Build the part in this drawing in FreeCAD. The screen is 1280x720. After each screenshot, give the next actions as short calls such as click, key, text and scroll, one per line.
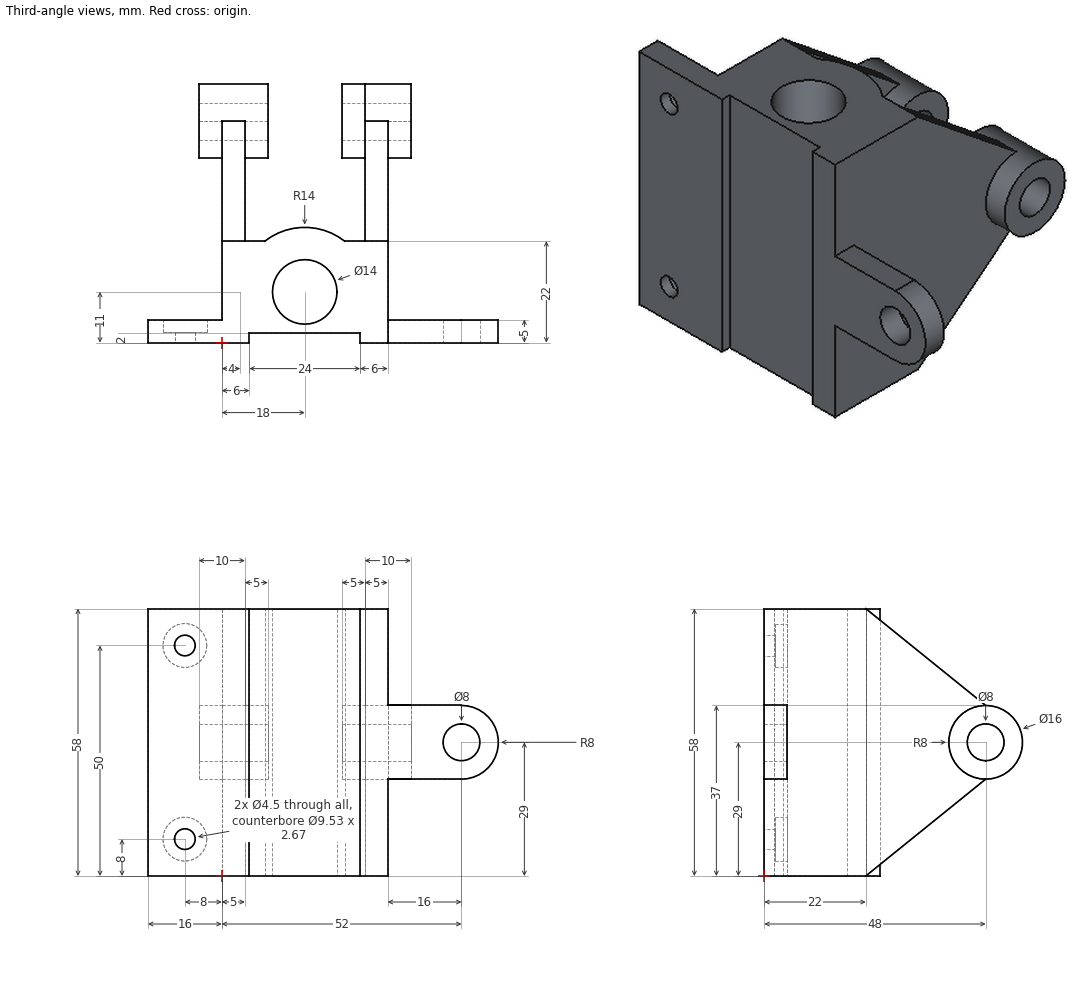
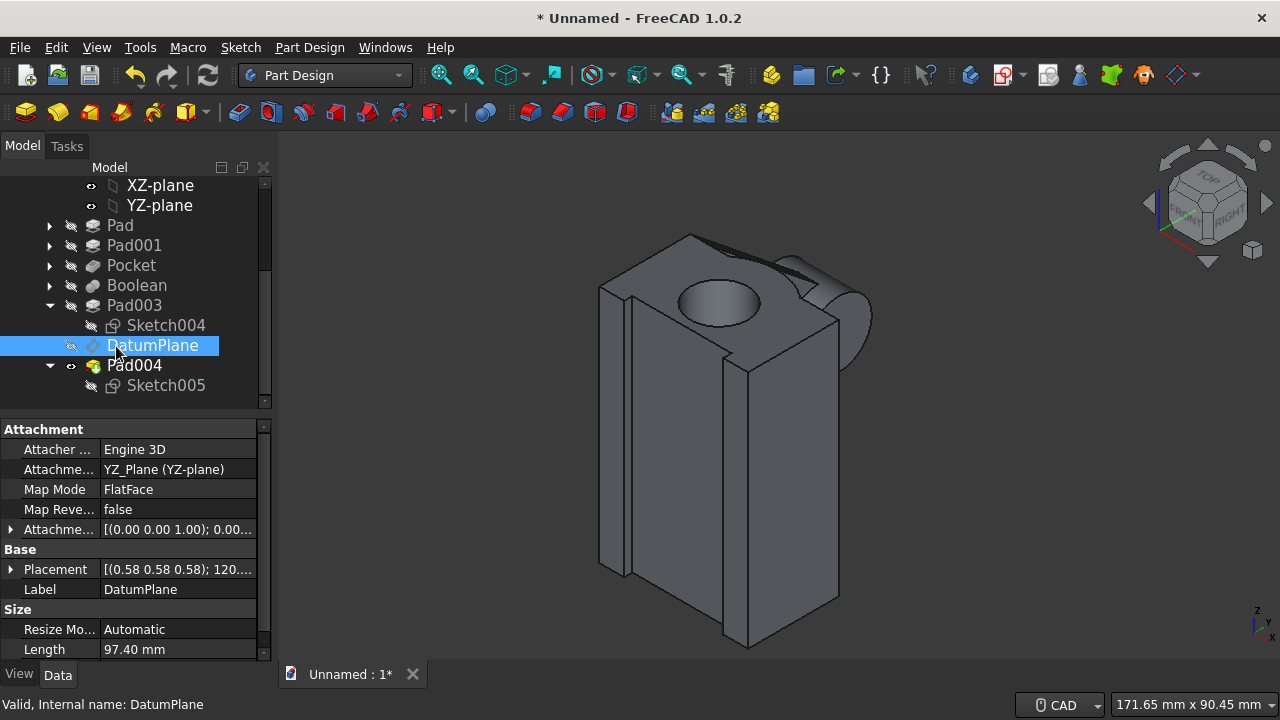
click(848, 328)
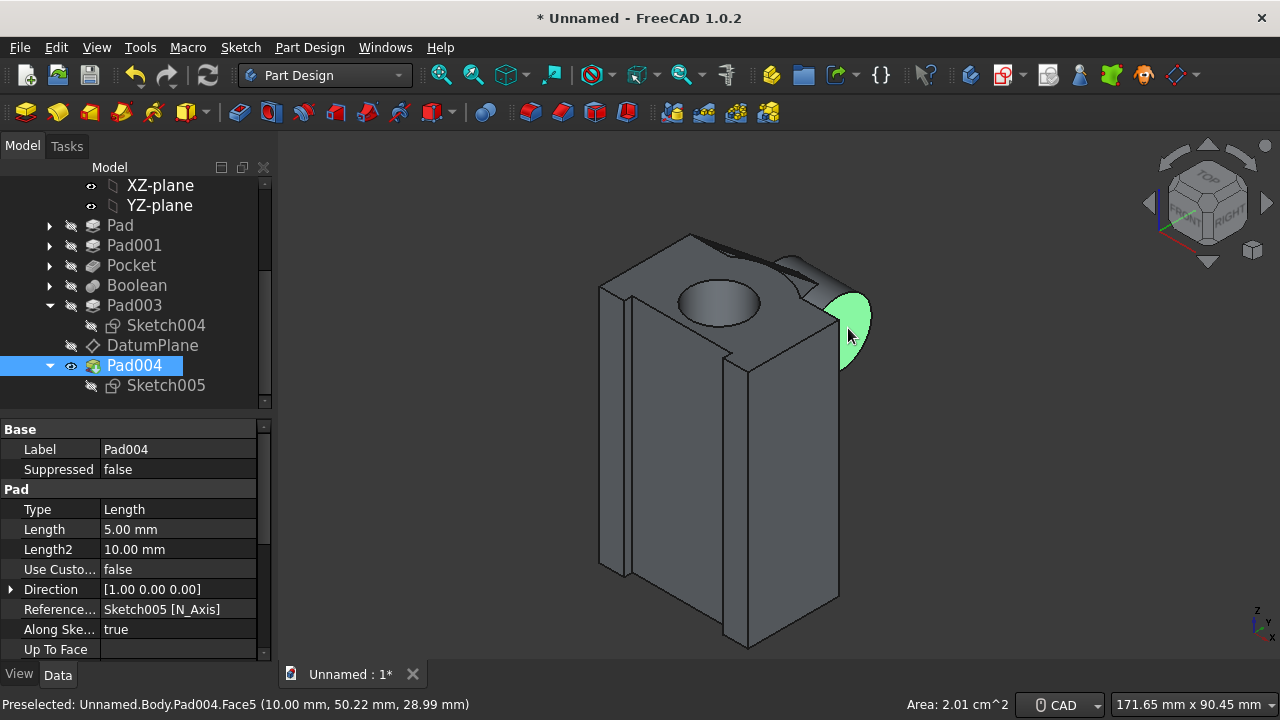
click(1004, 76)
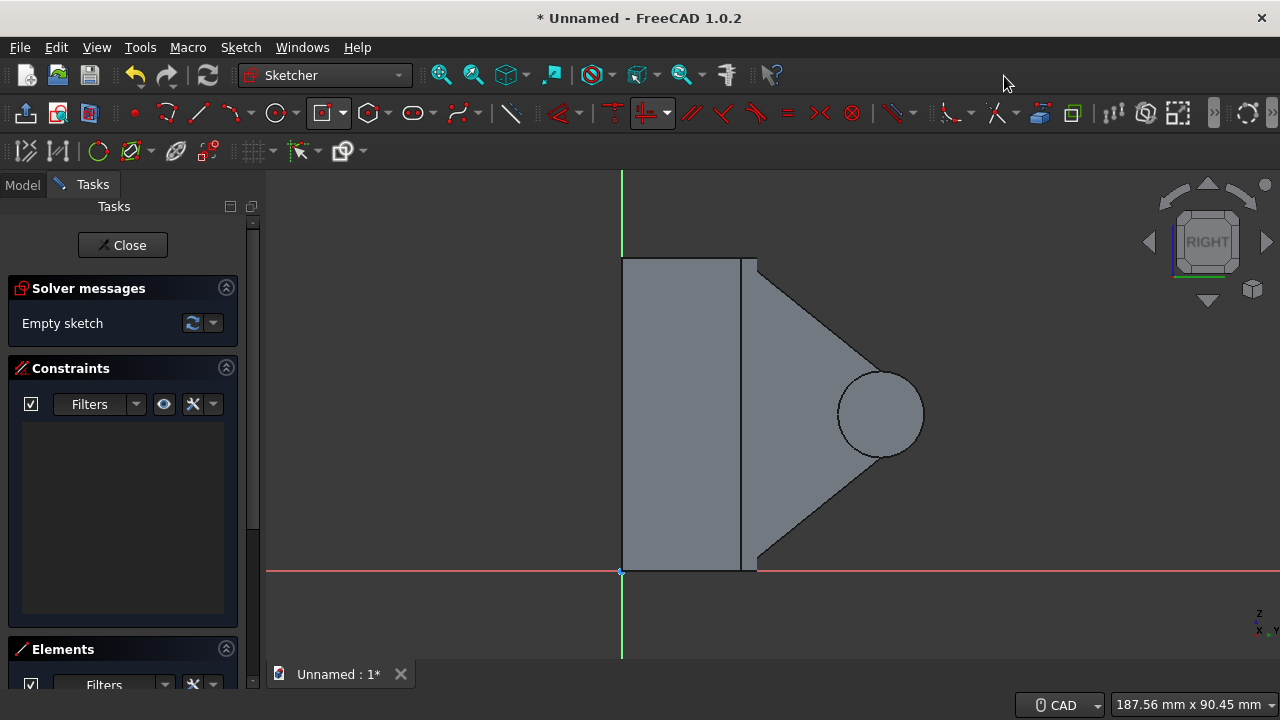
scroll(909, 414, up, 10)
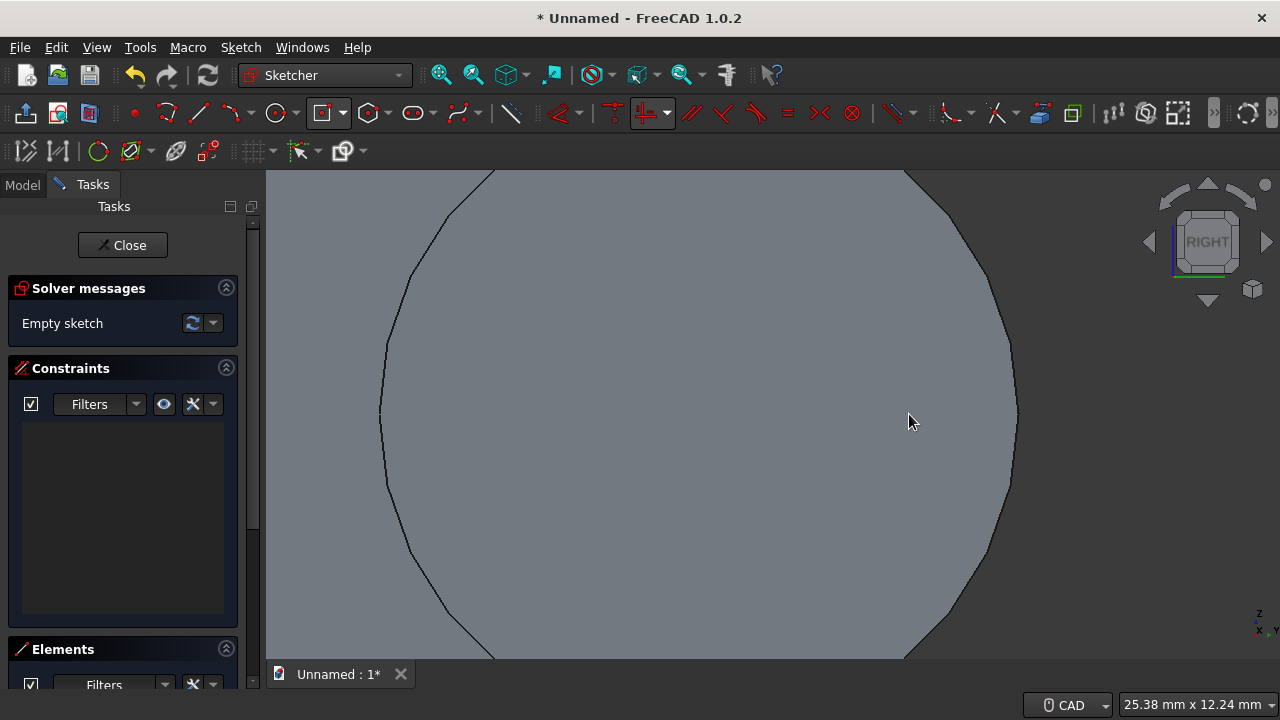
key(g)
key(c)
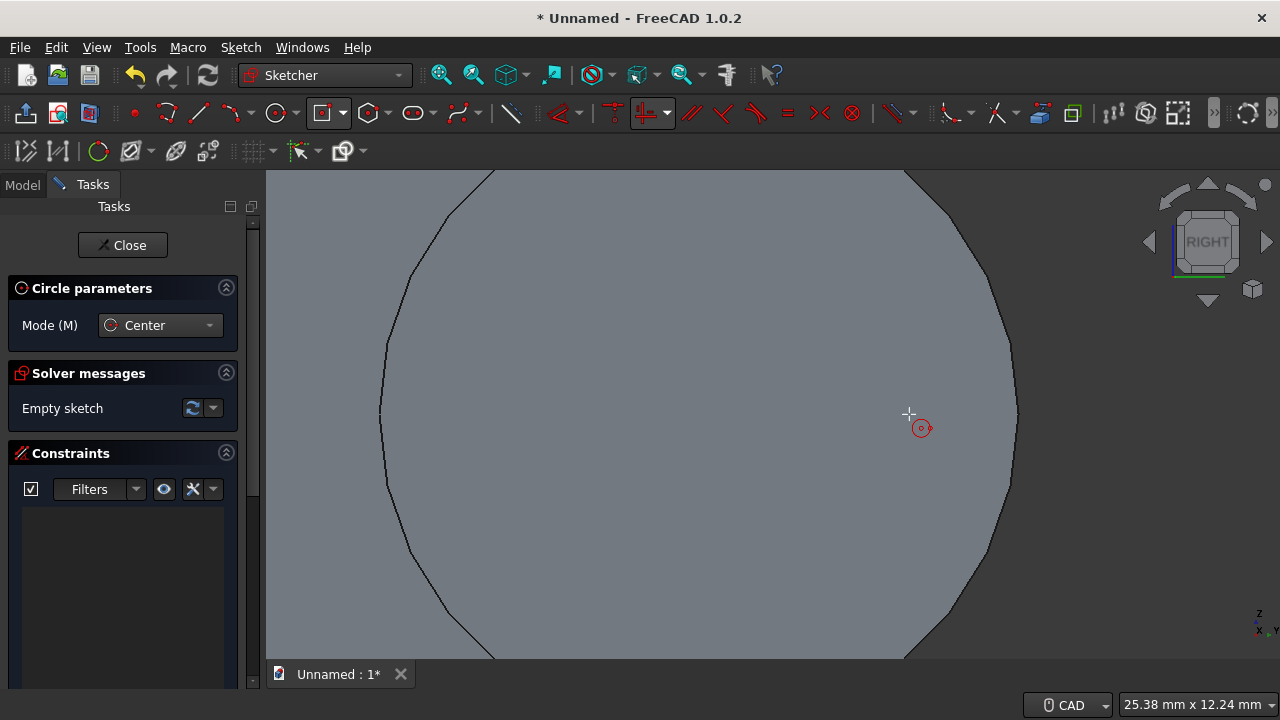
click(699, 414)
move(812, 302)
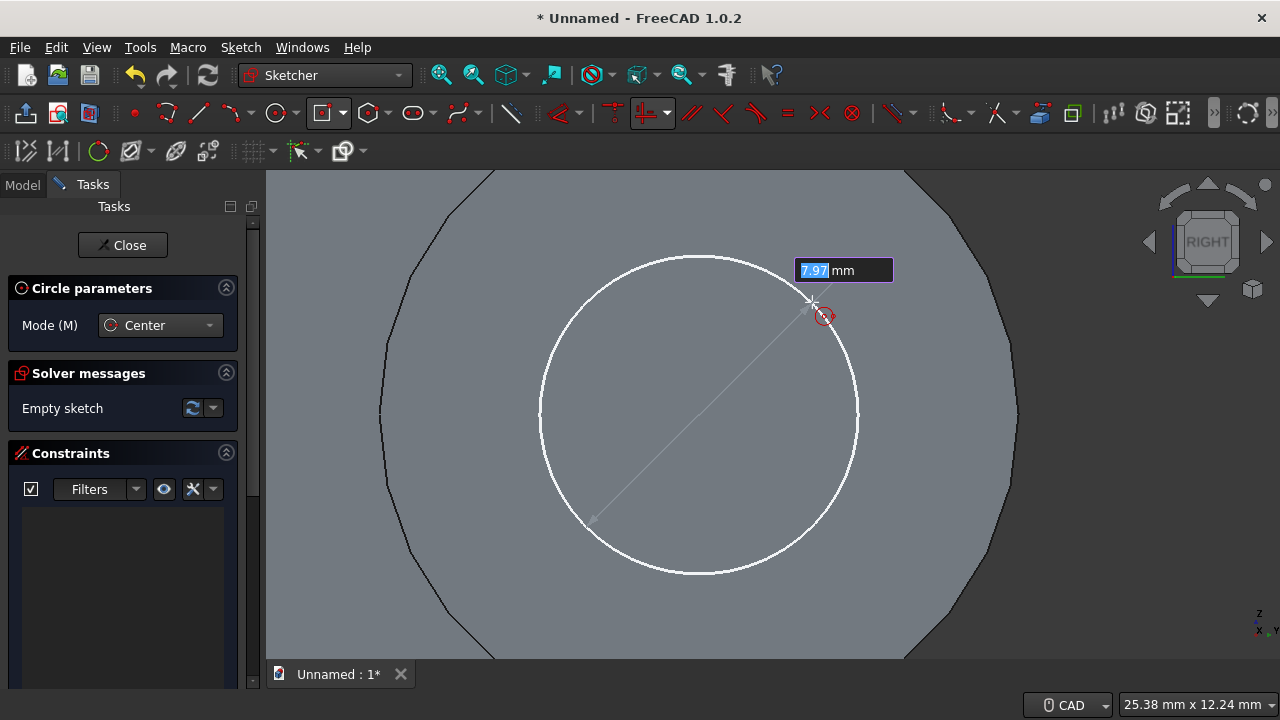
text(8)
key(Return)
key(Escape)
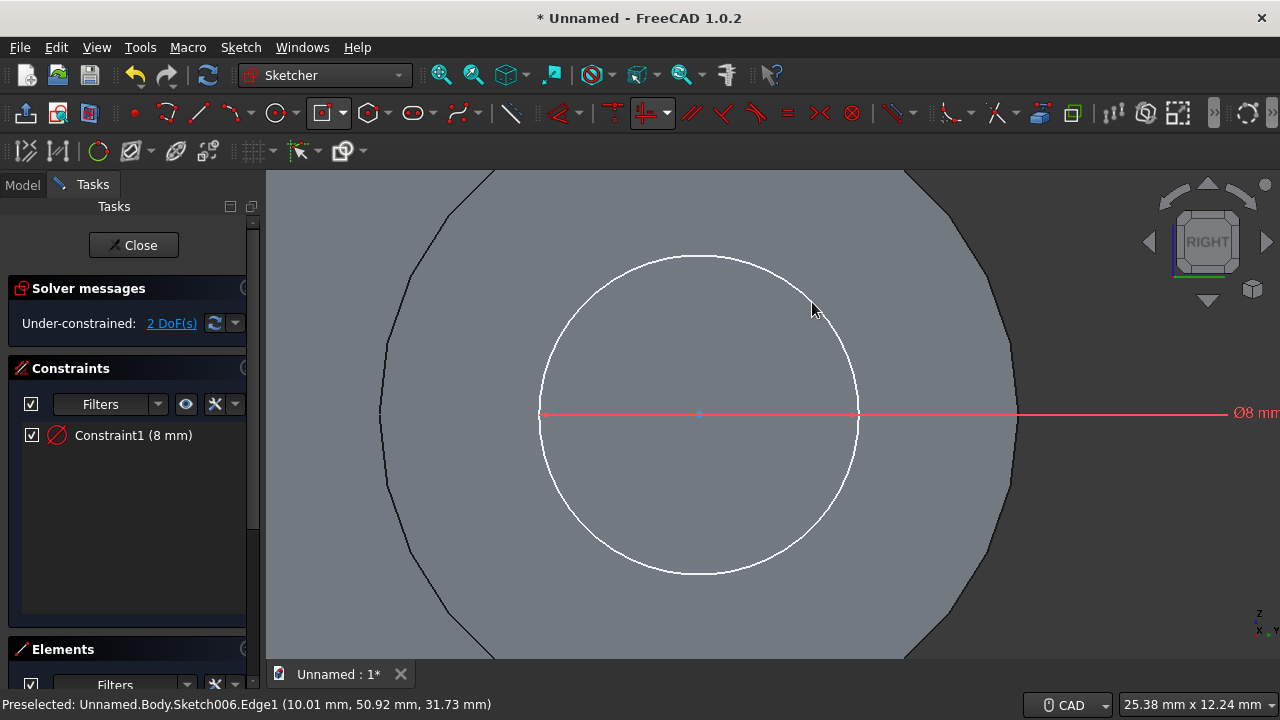
click(558, 114)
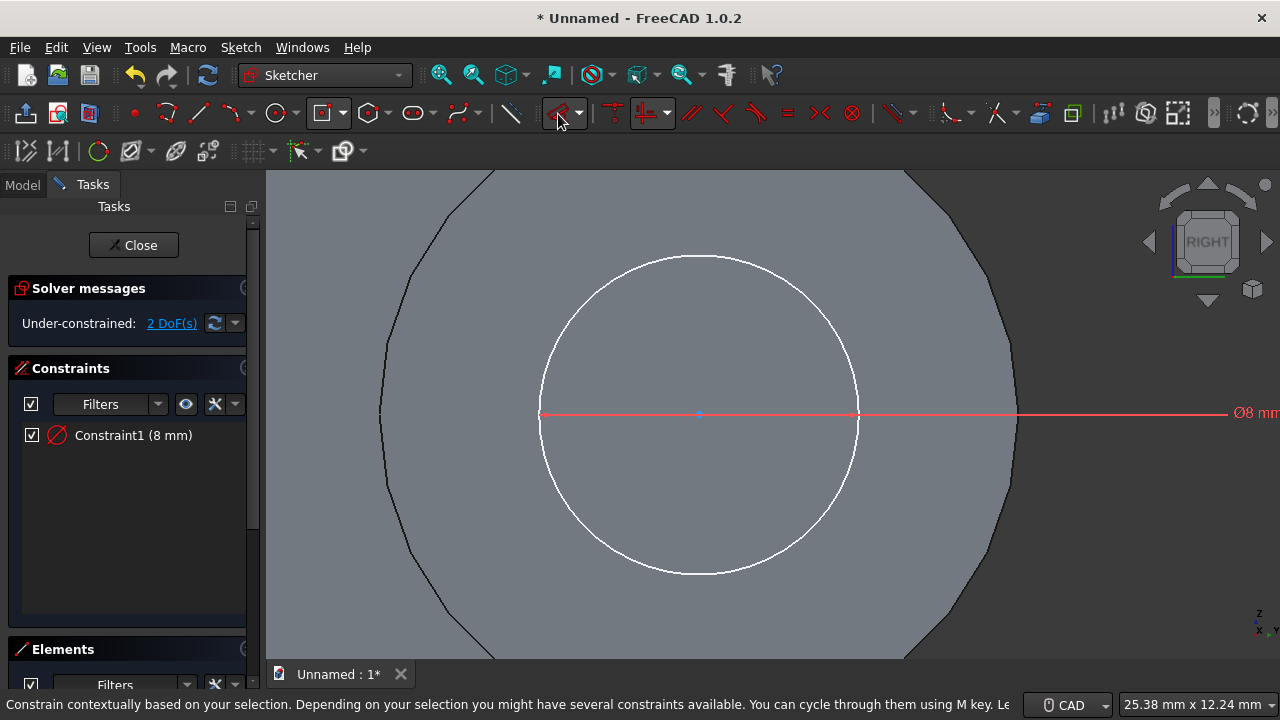
click(699, 415)
click(497, 381)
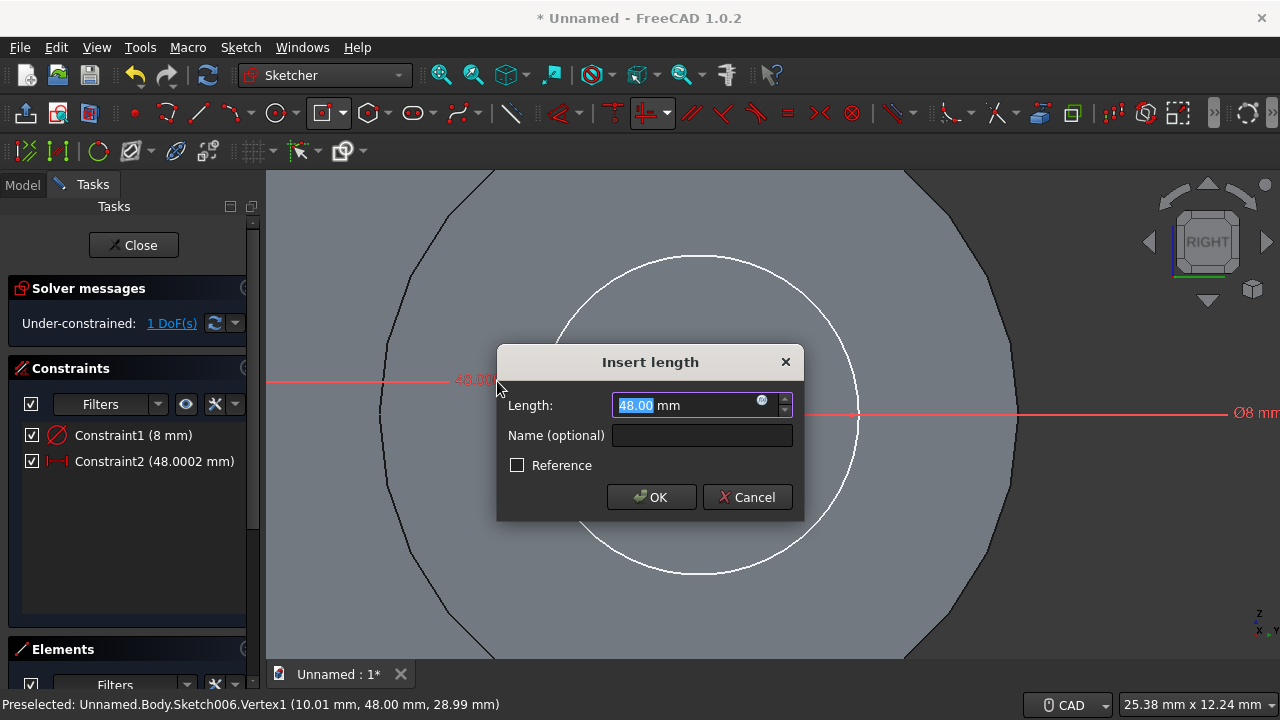
text(48)
key(Return)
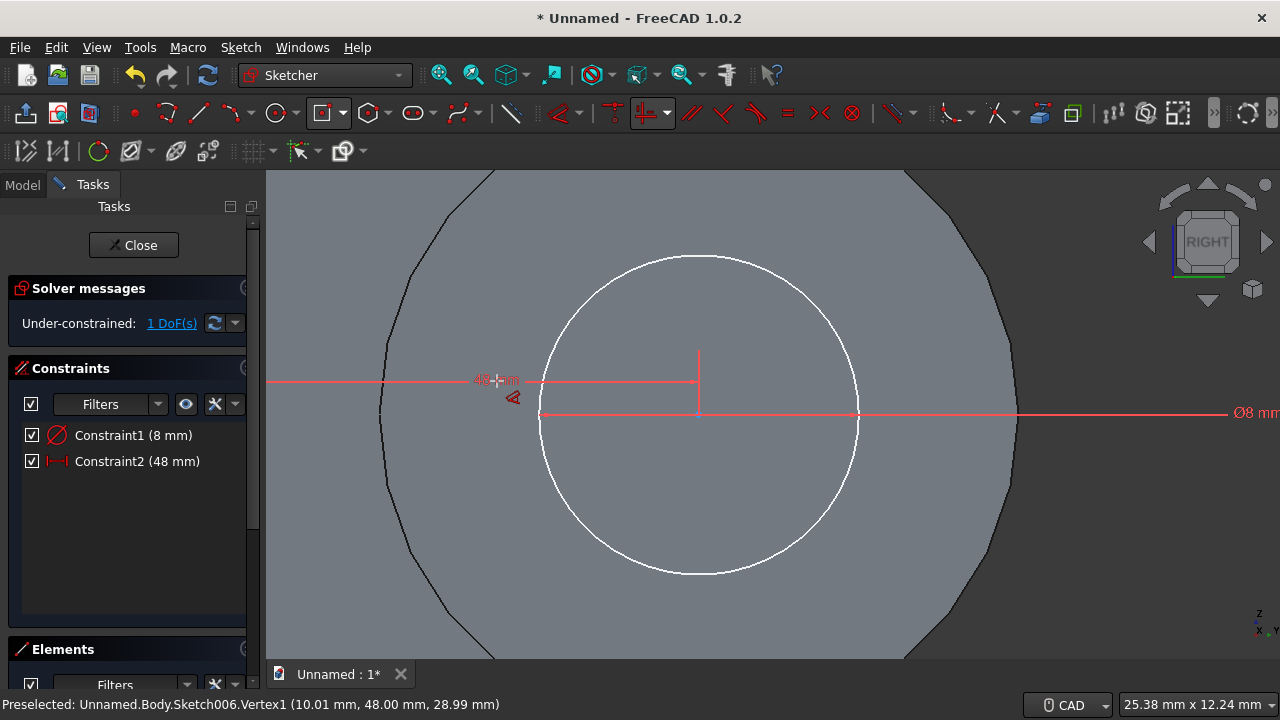
click(699, 415)
click(733, 523)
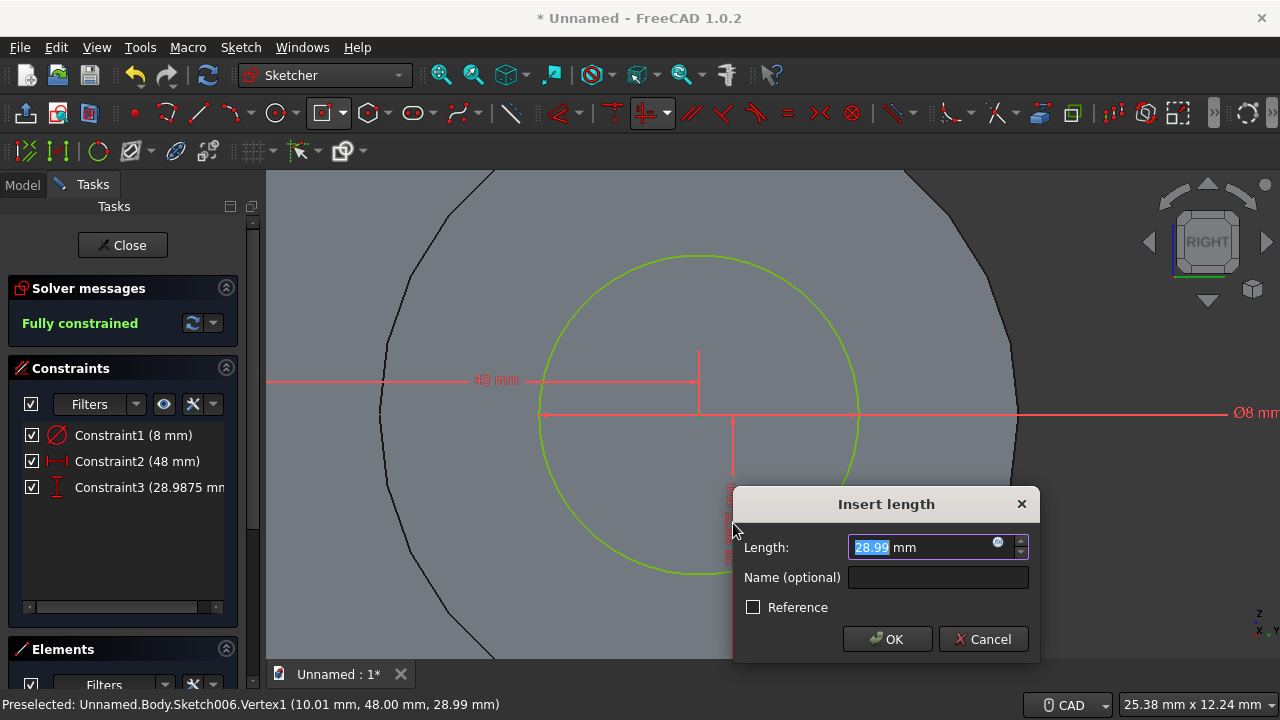
text(29)
key(Return)
key(Escape)